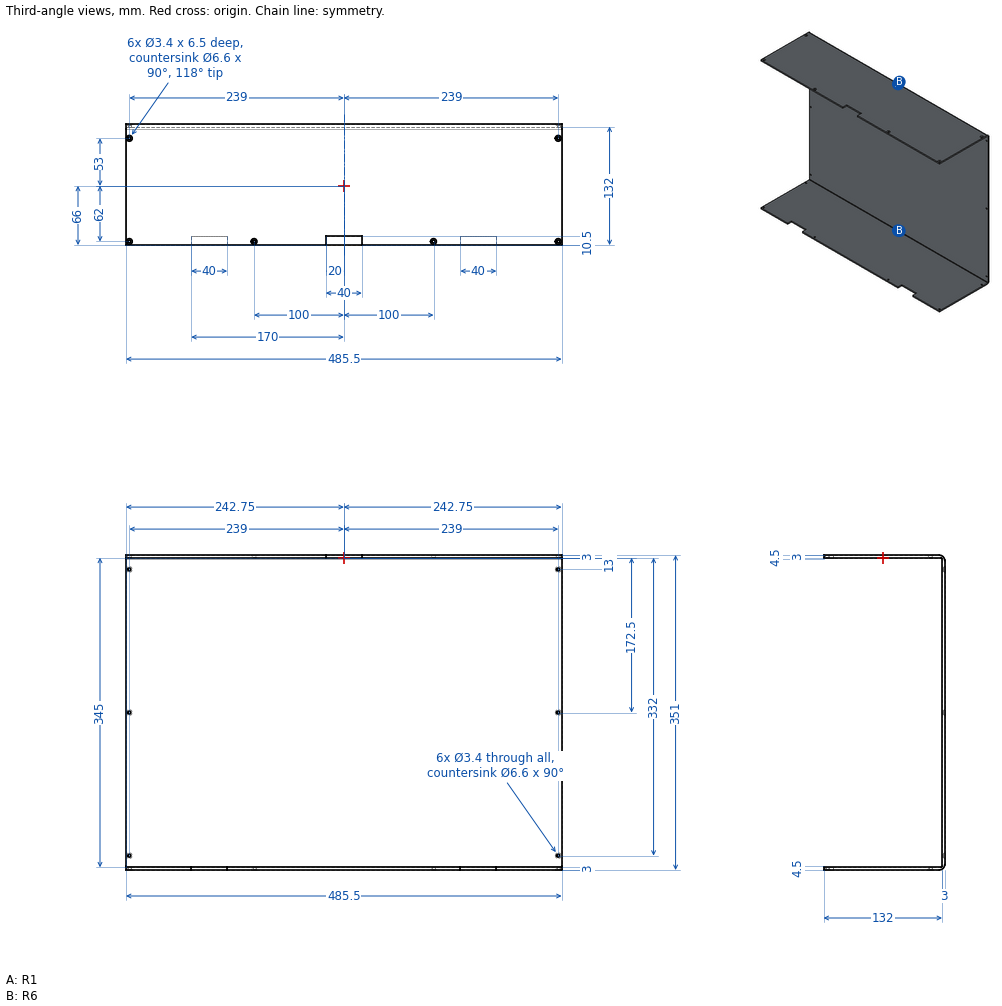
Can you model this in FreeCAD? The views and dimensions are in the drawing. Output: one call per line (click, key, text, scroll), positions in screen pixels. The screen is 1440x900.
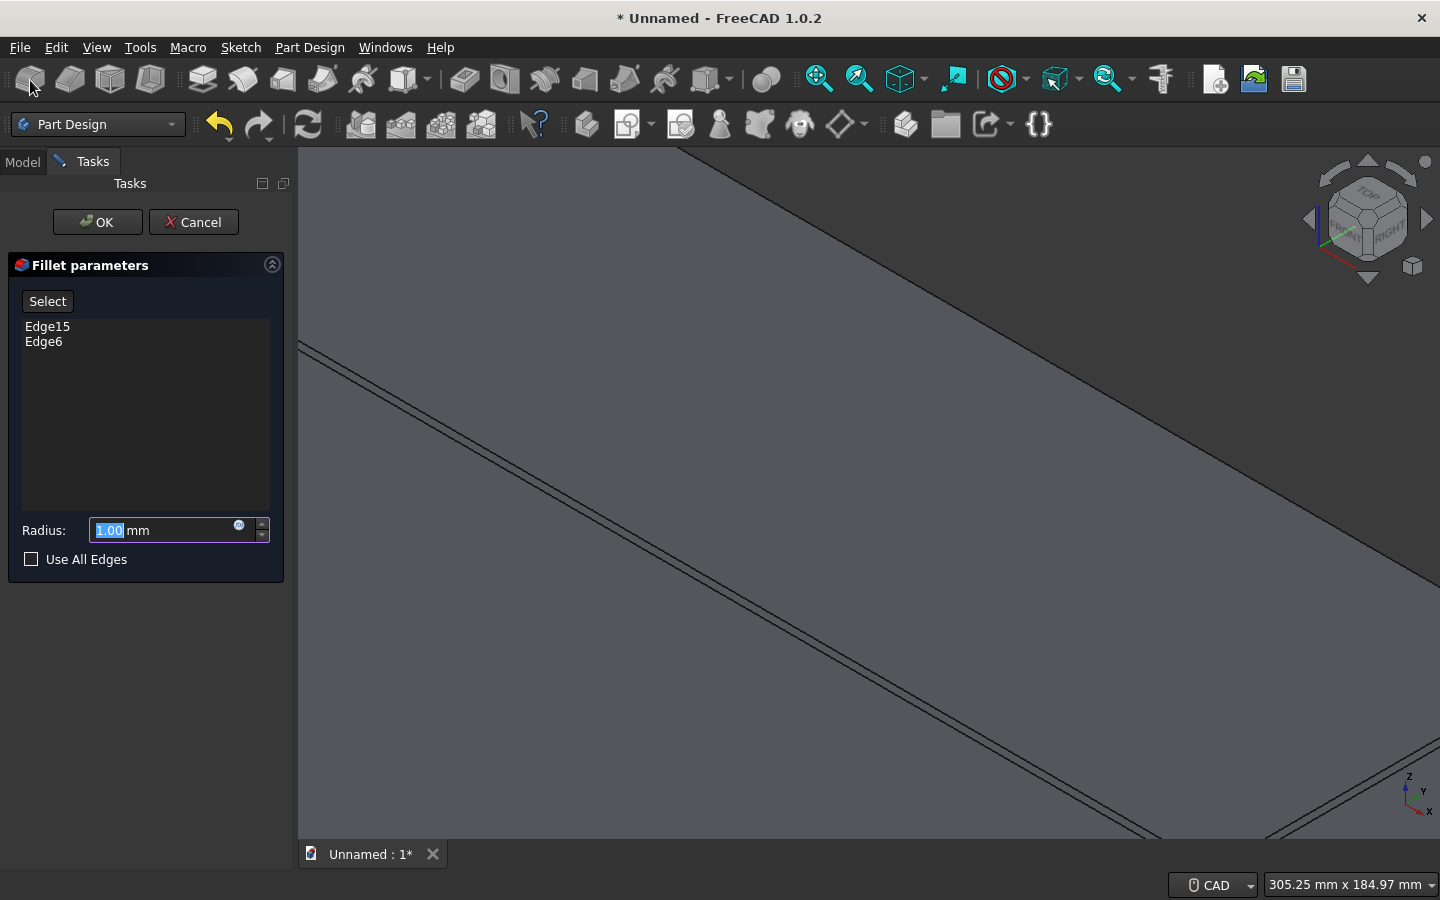
text(1)
key(Tab)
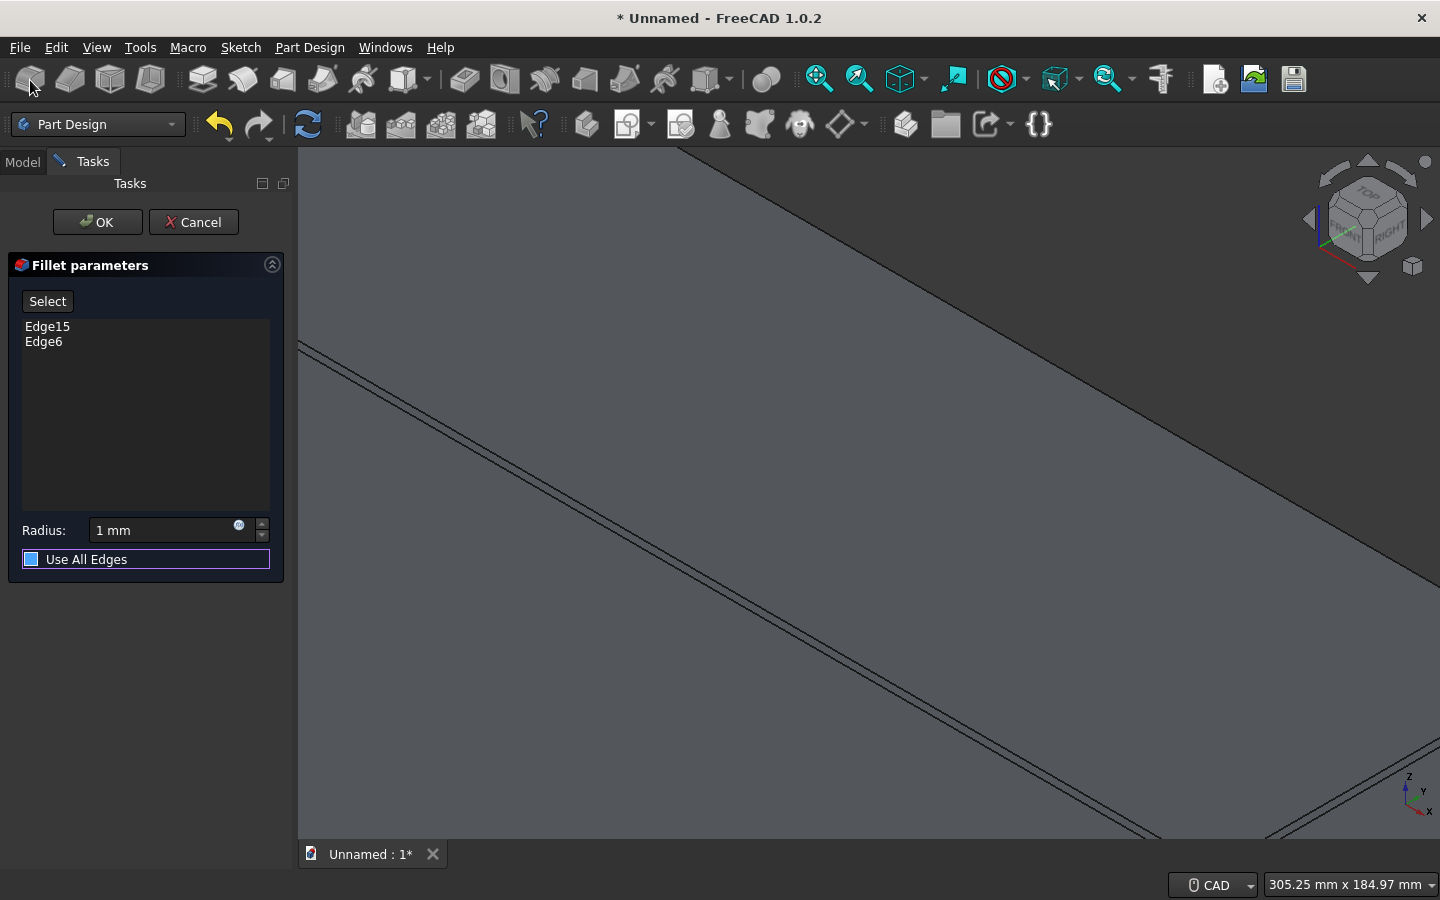
click(98, 222)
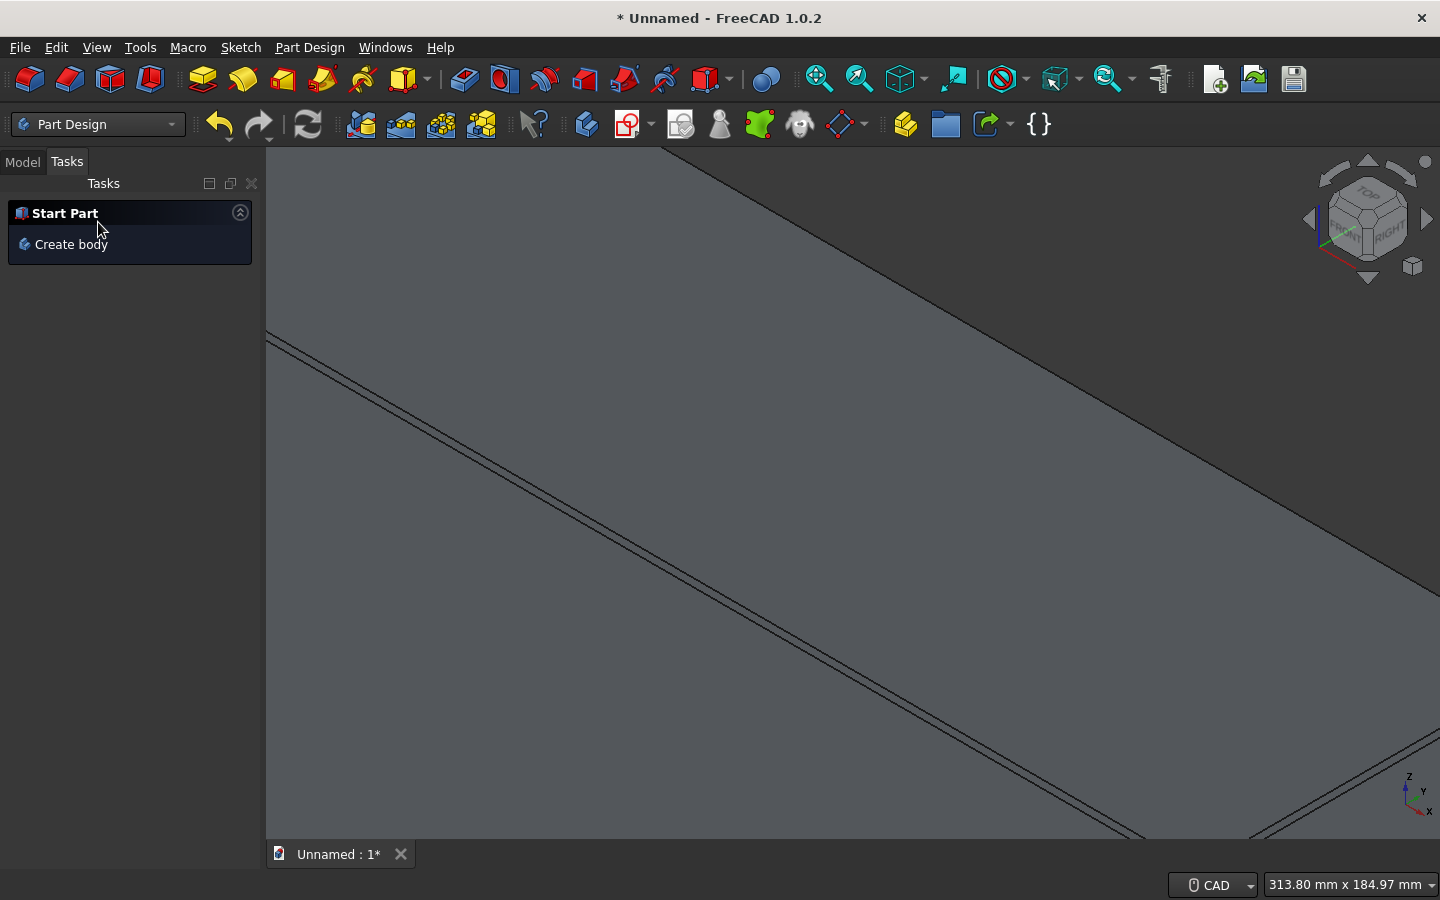
click(820, 80)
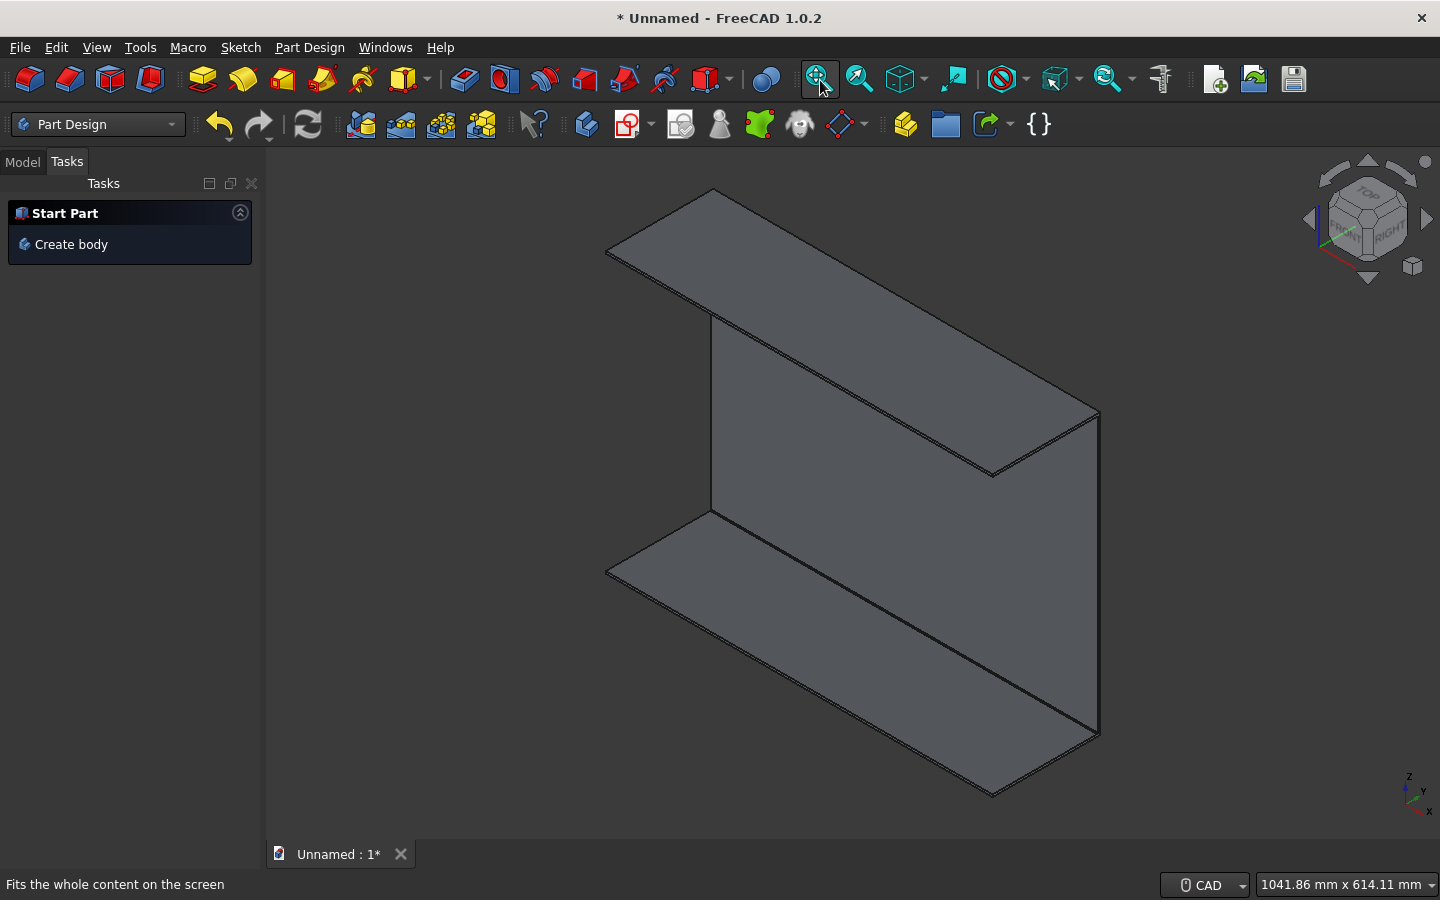
key(2)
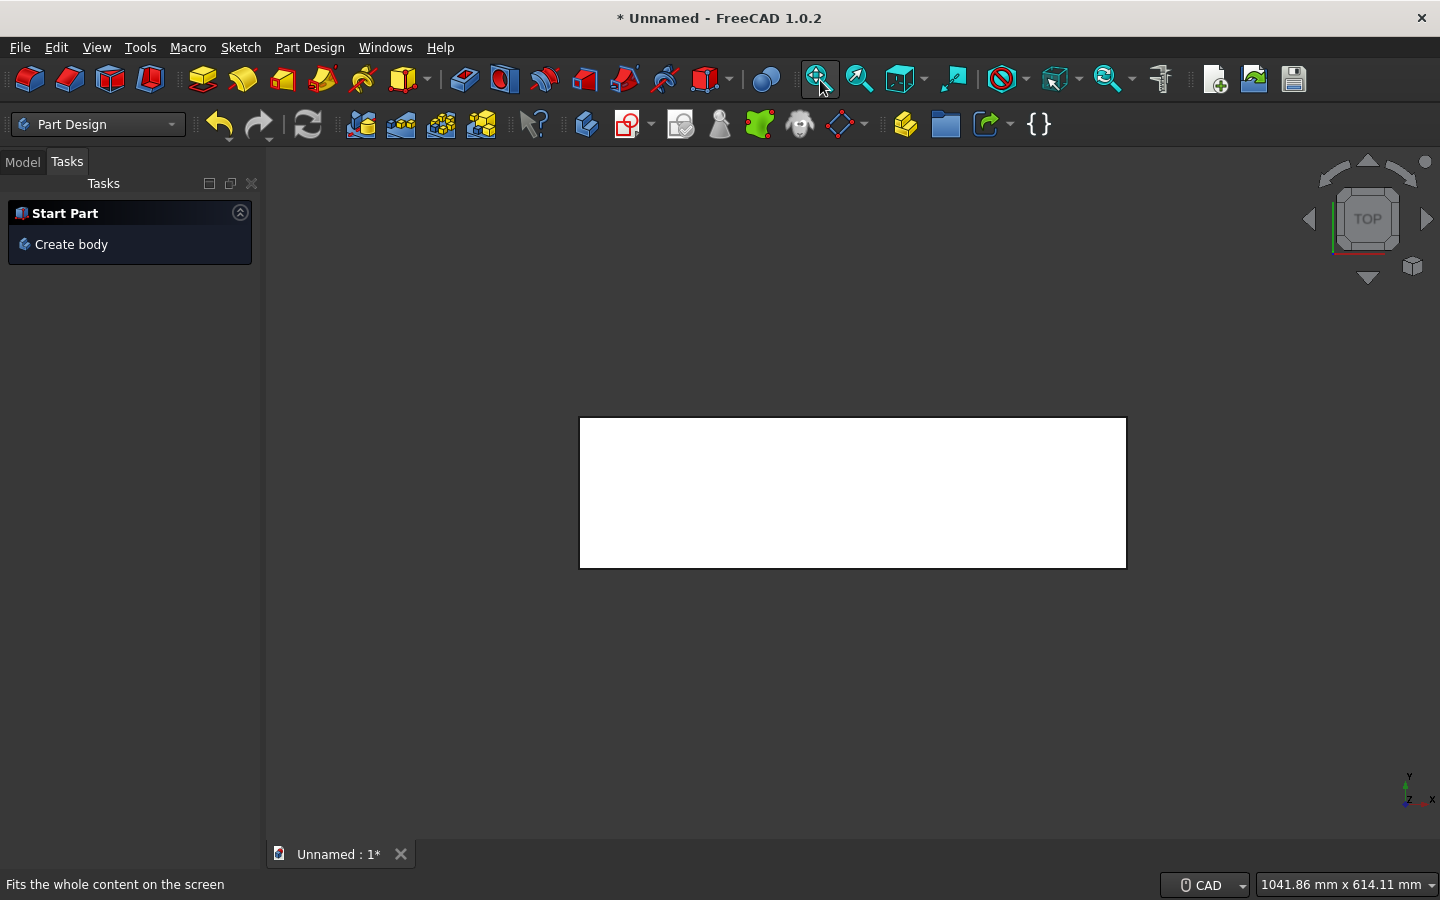
click(853, 416)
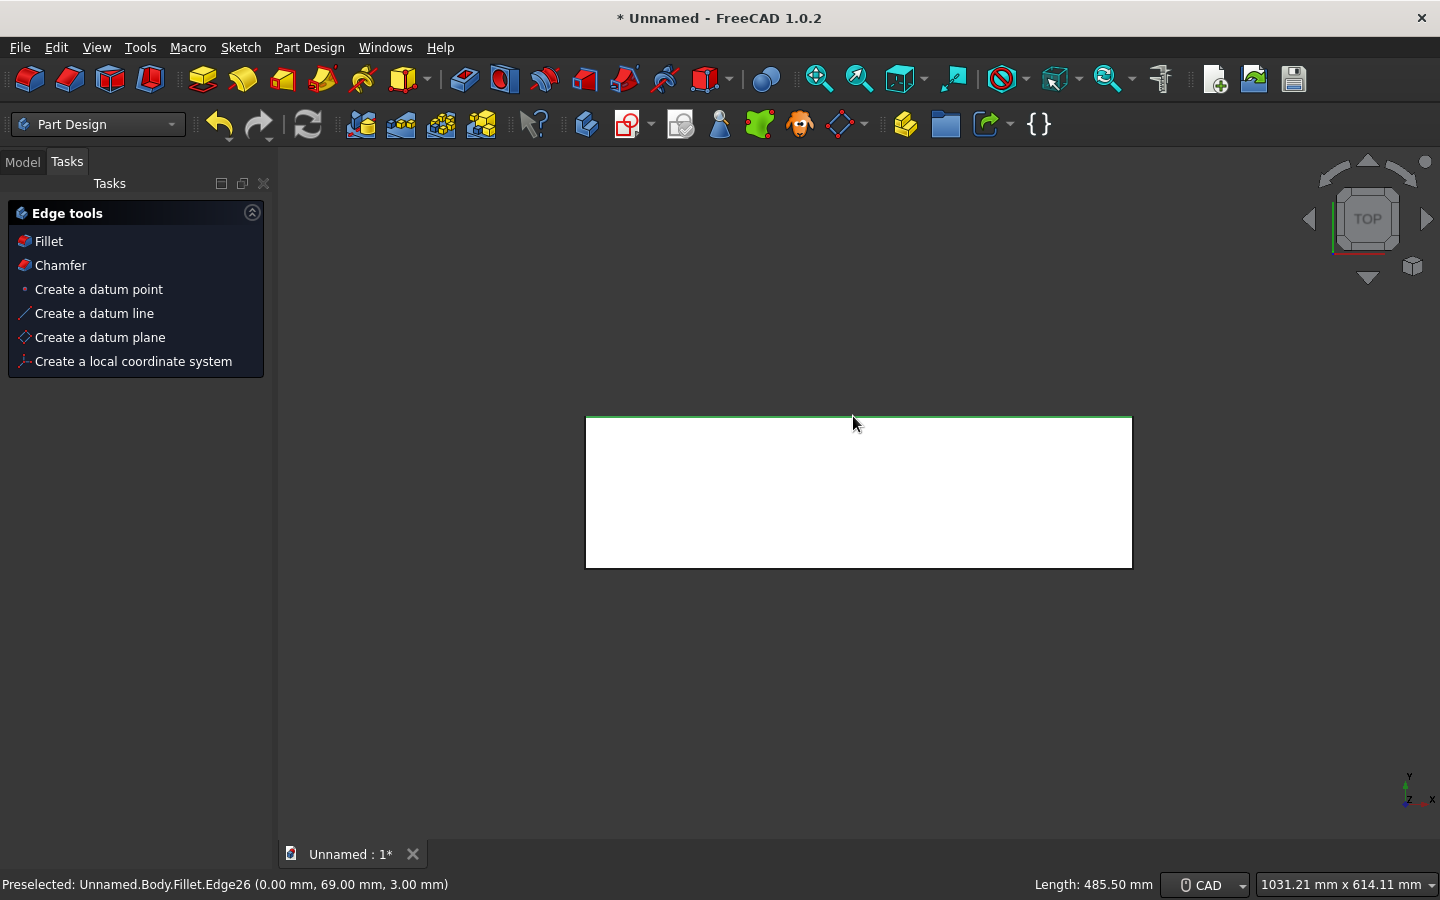
key(0)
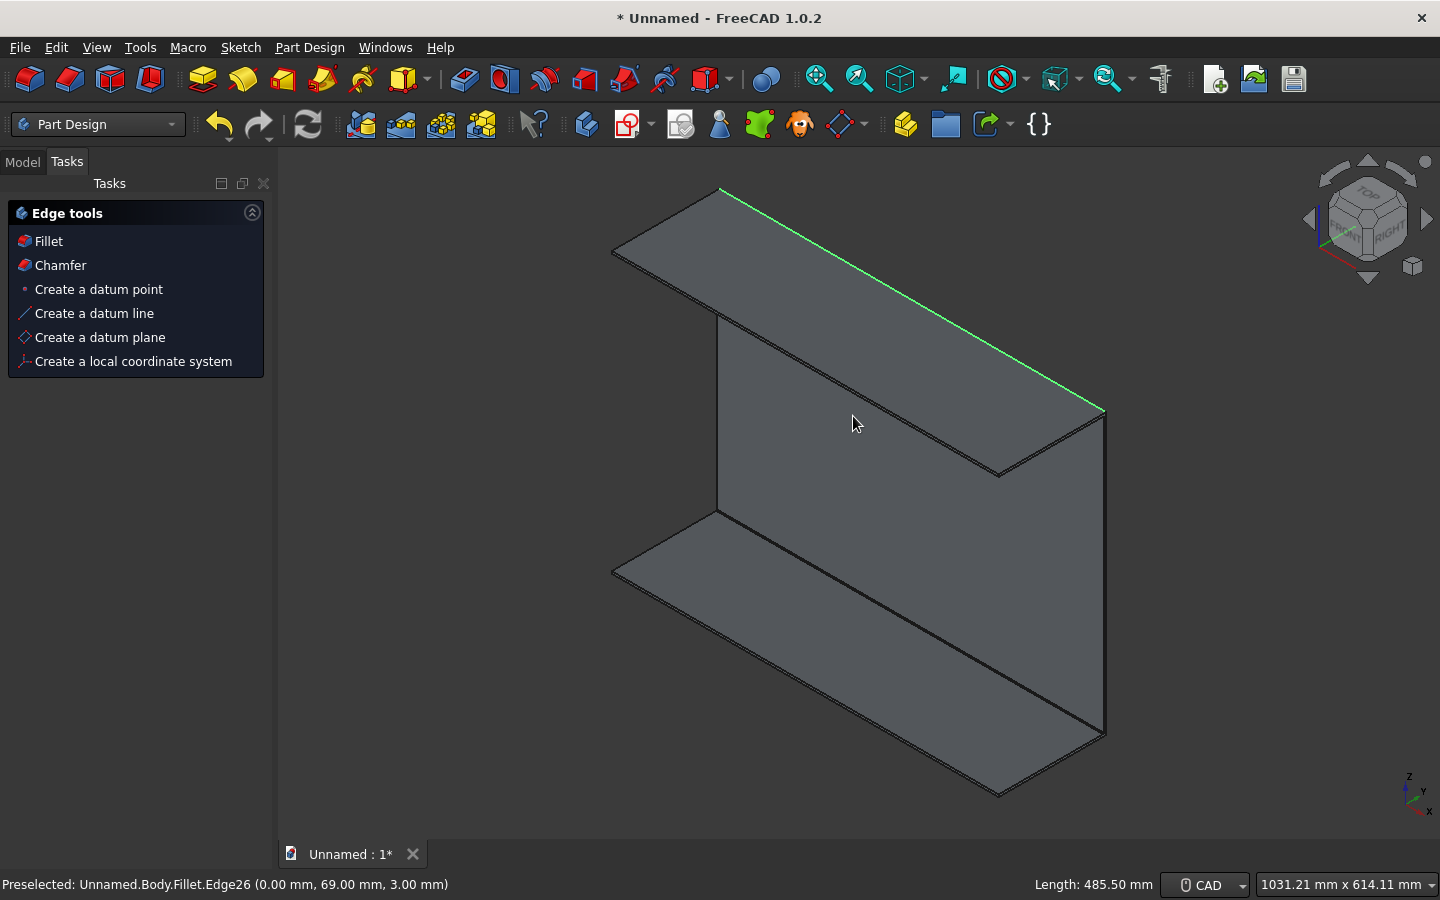
key(1)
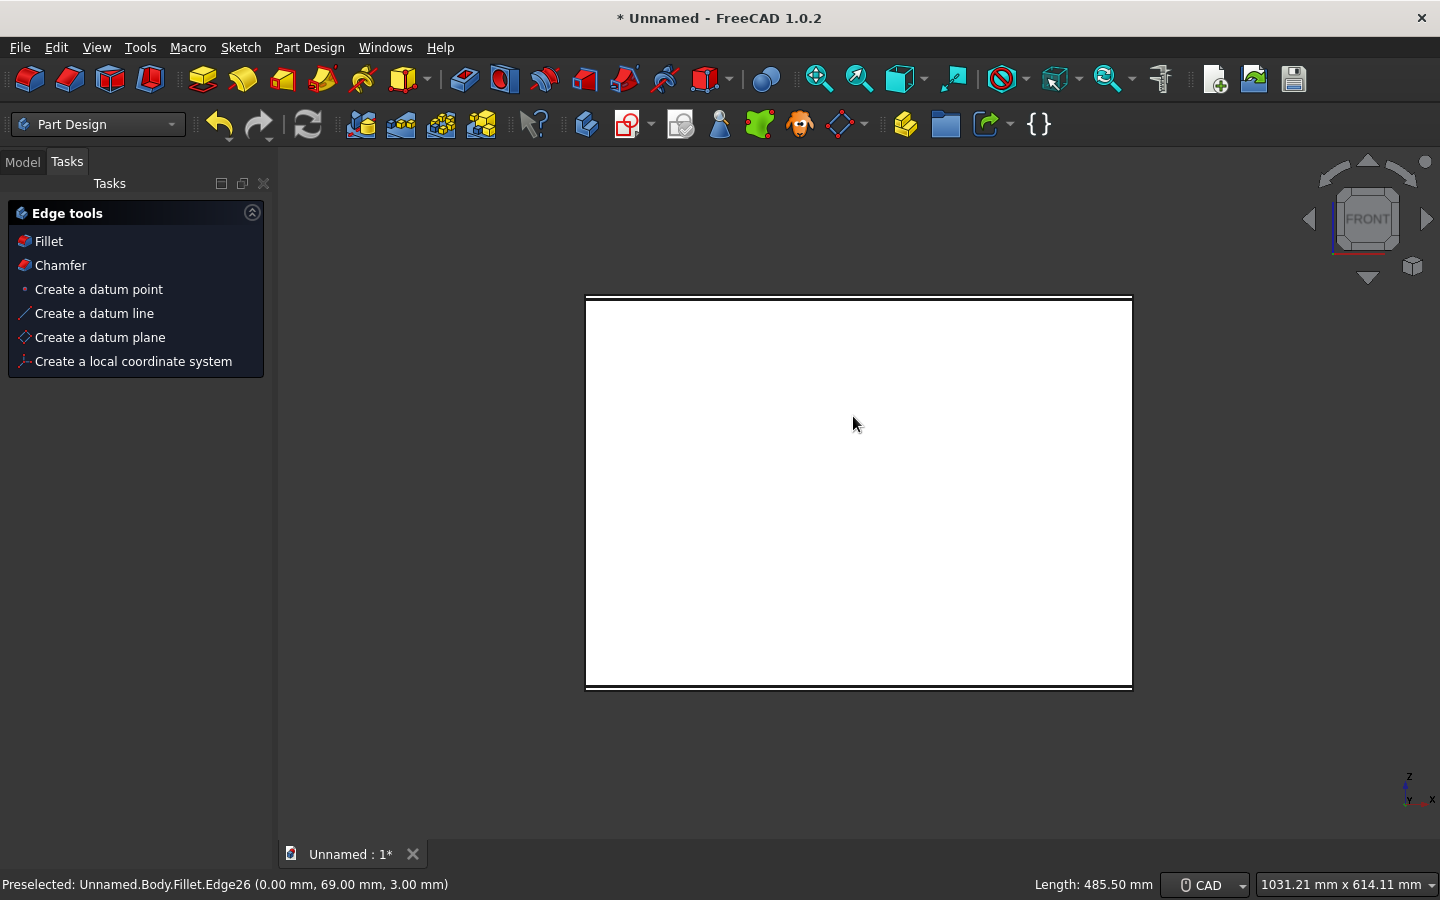
key(3)